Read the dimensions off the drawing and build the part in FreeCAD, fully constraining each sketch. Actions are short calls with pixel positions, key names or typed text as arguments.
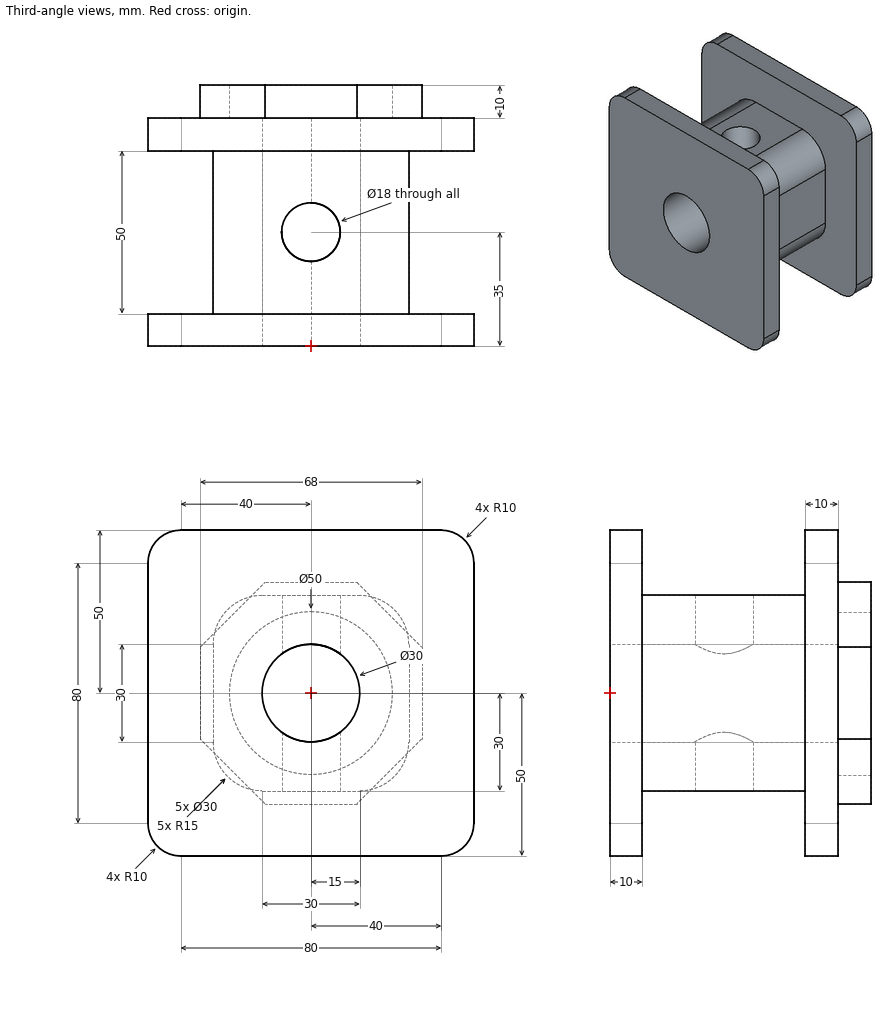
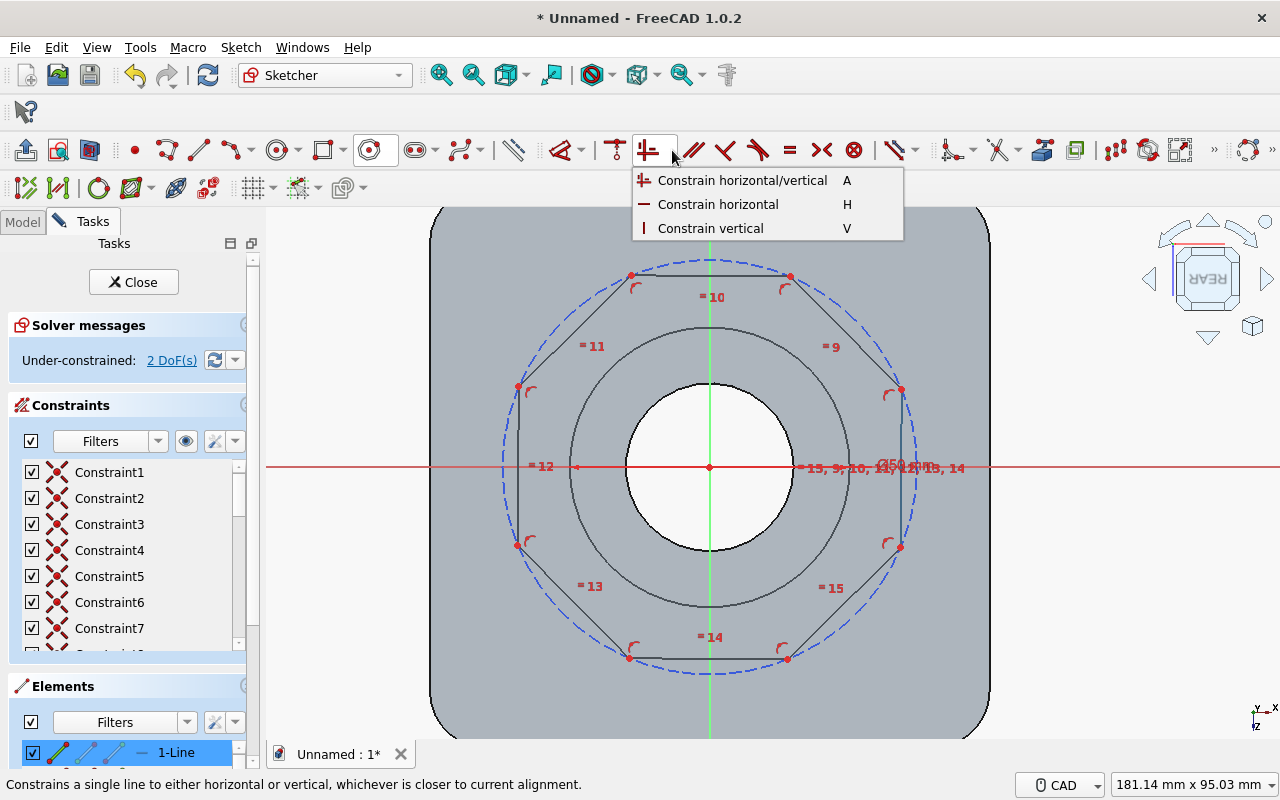
click(768, 228)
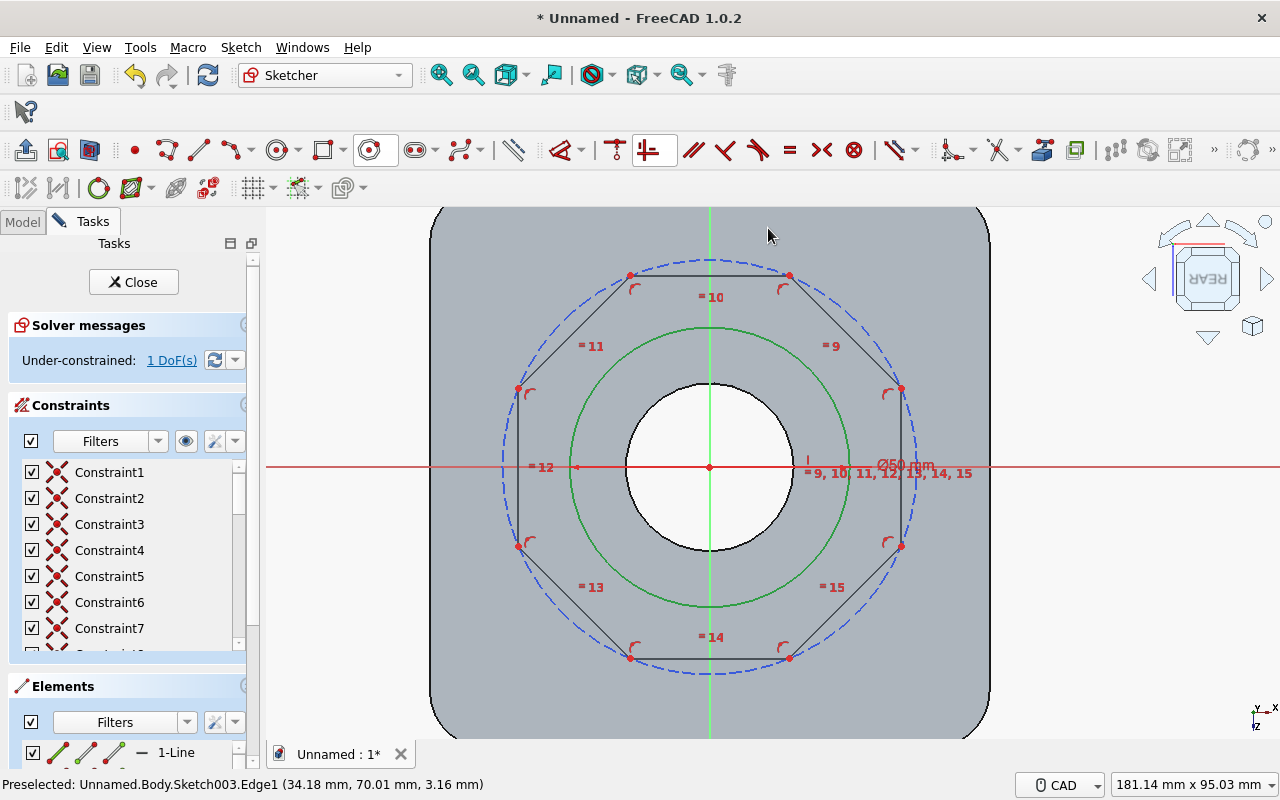
click(560, 150)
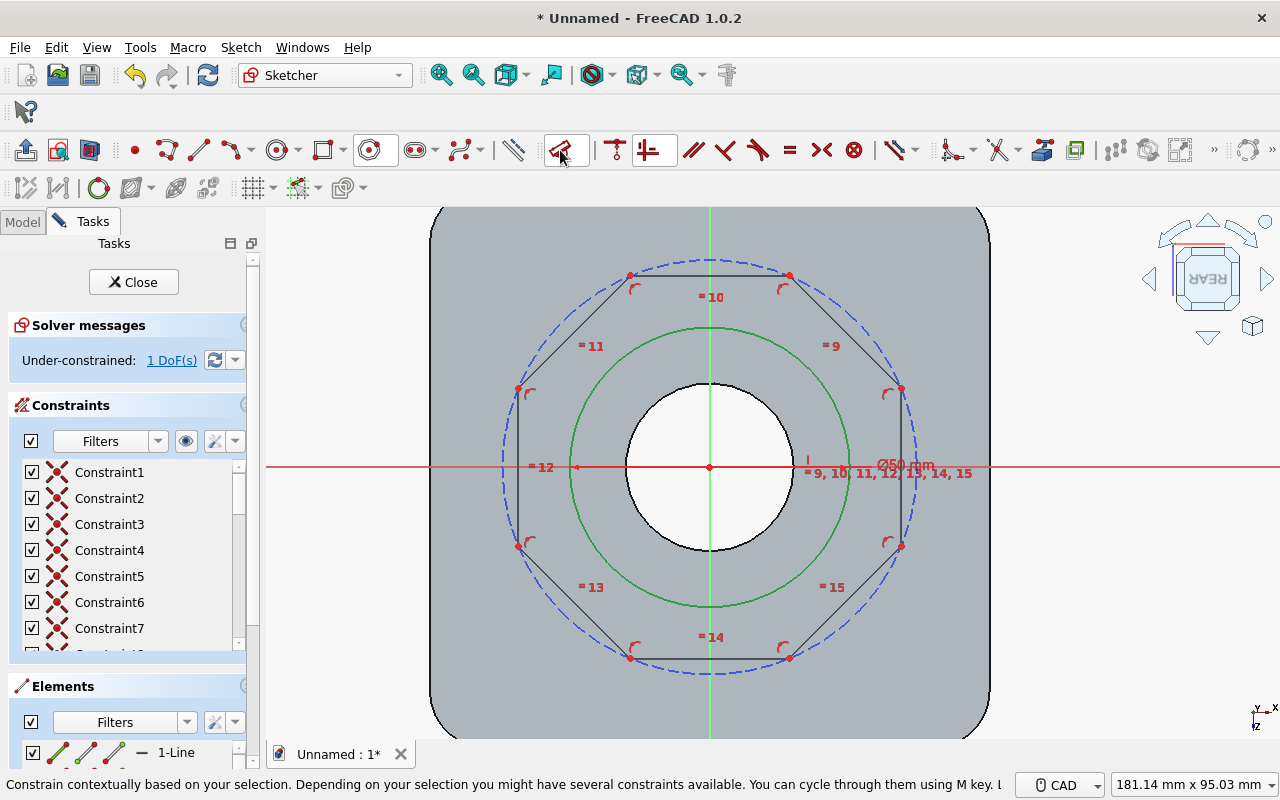
click(518, 388)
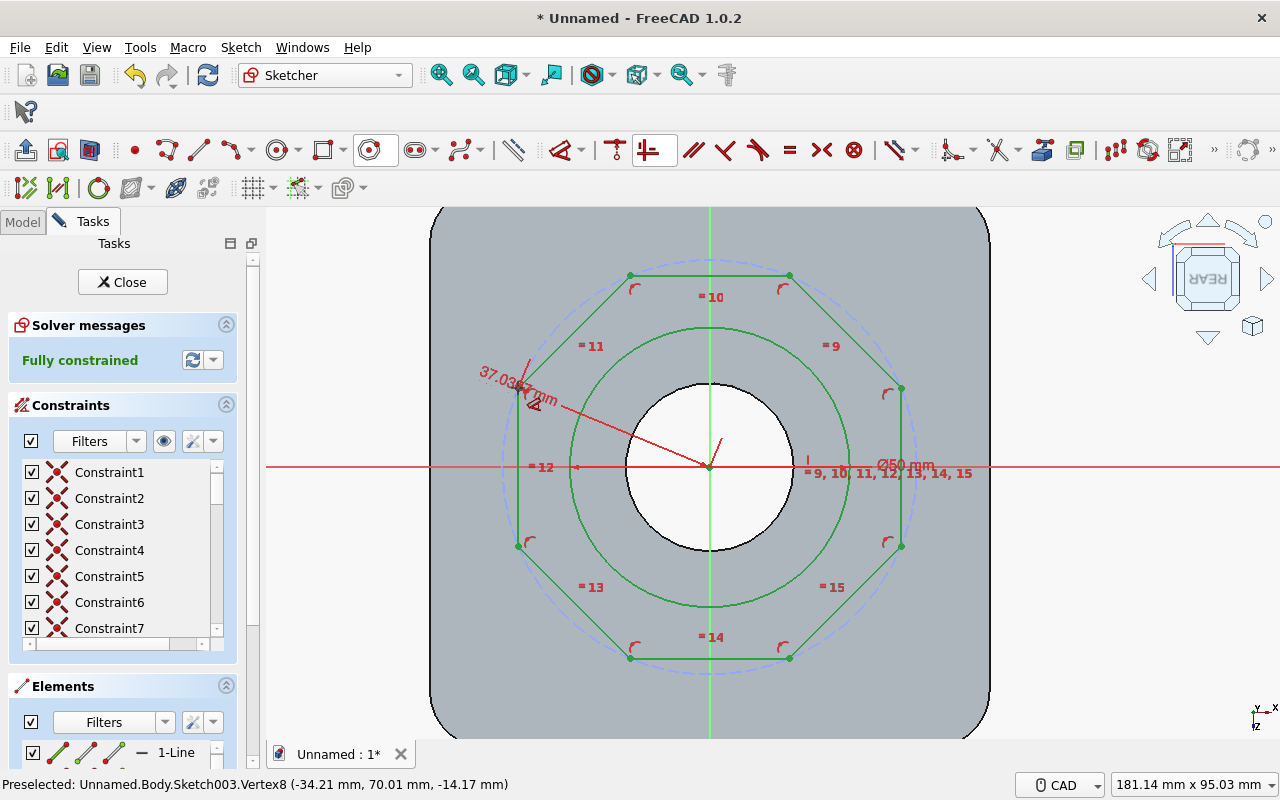
click(901, 547)
click(576, 581)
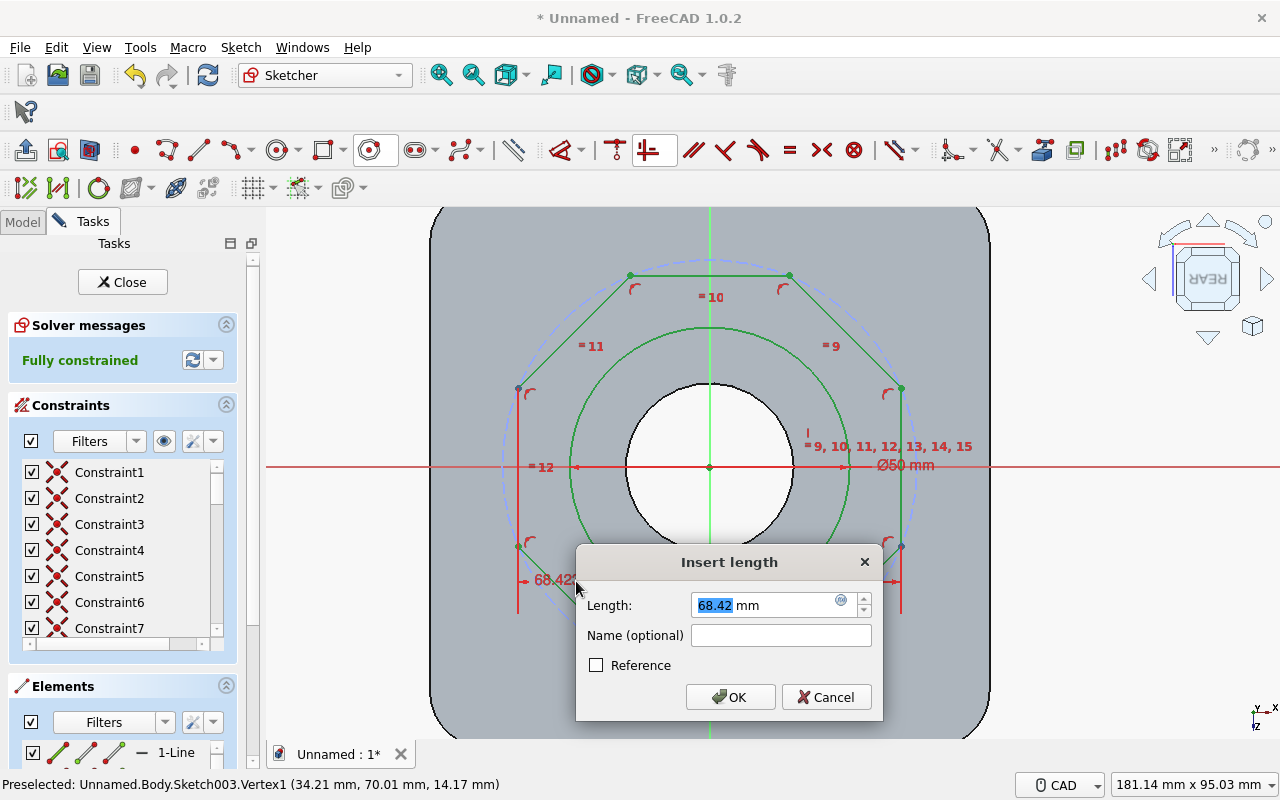
text(68)
key(Return)
key(Escape)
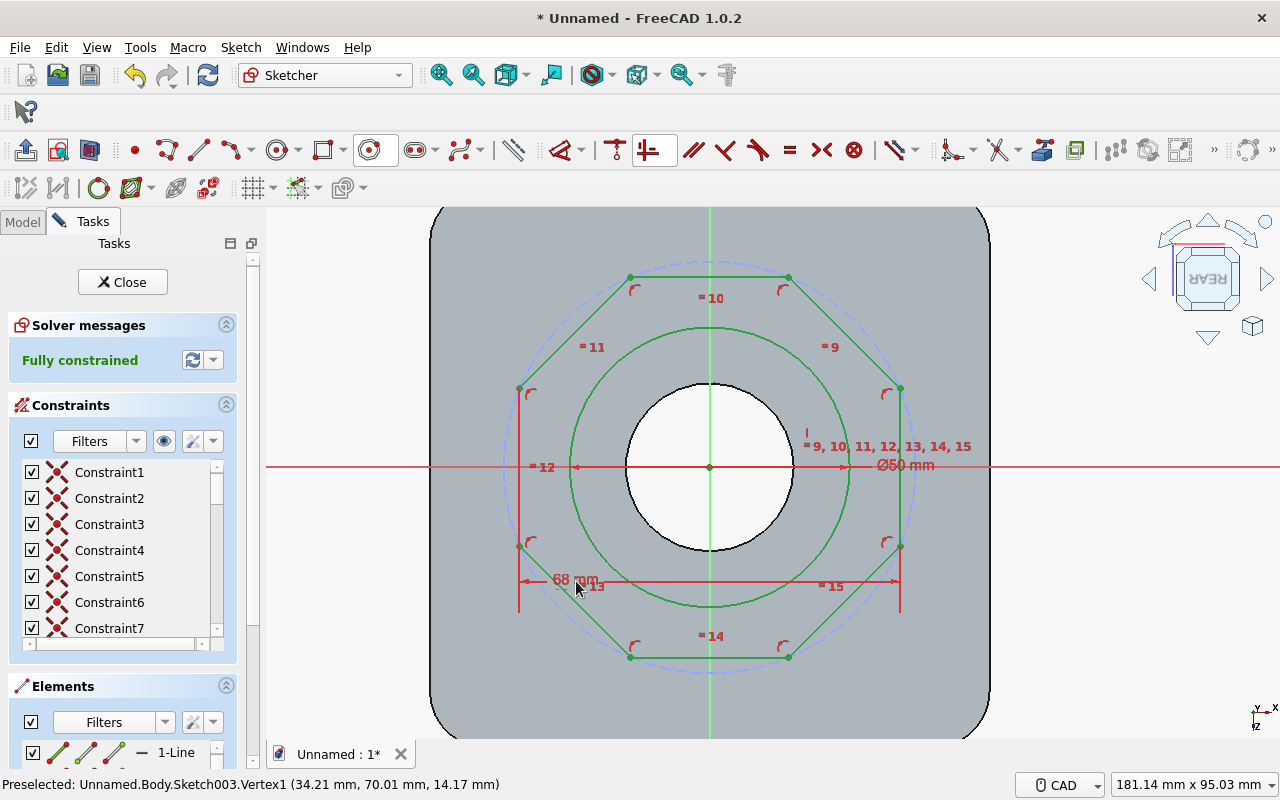
click(123, 282)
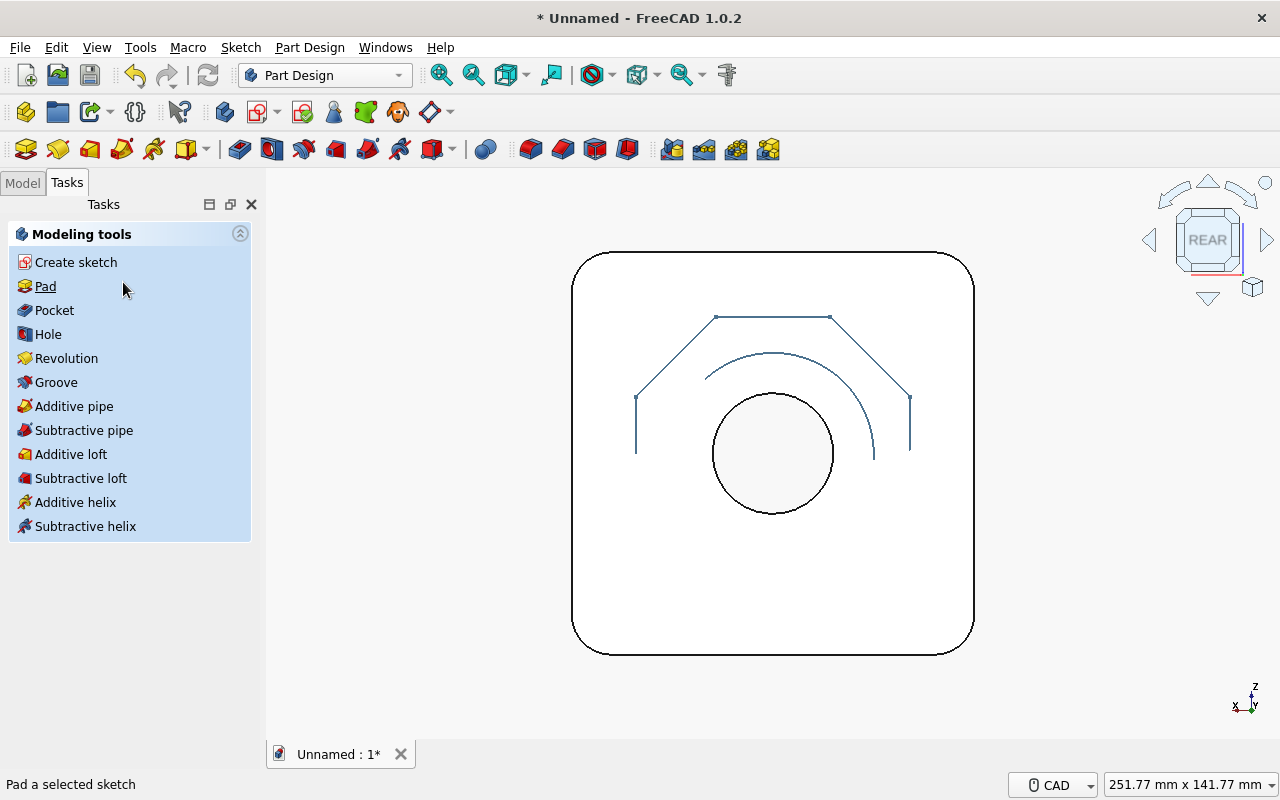
click(26, 150)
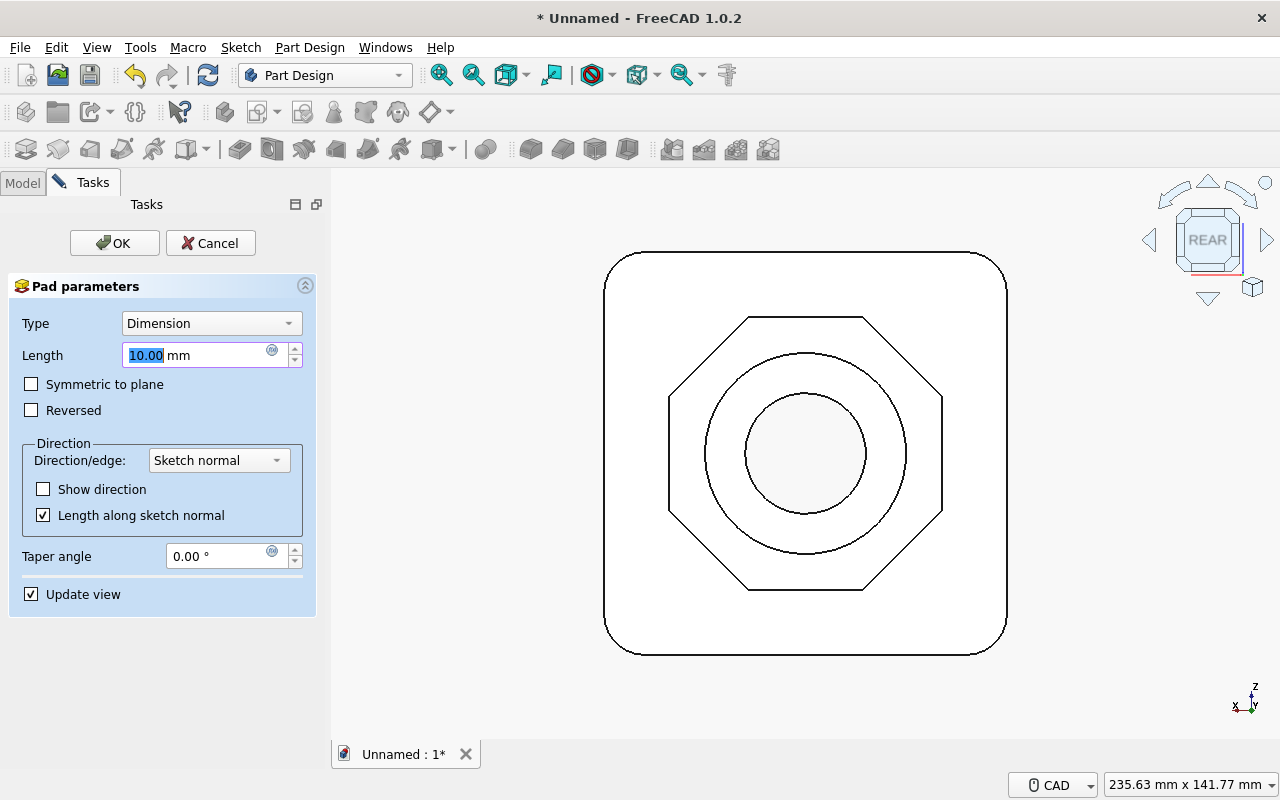
text(10)
key(Tab)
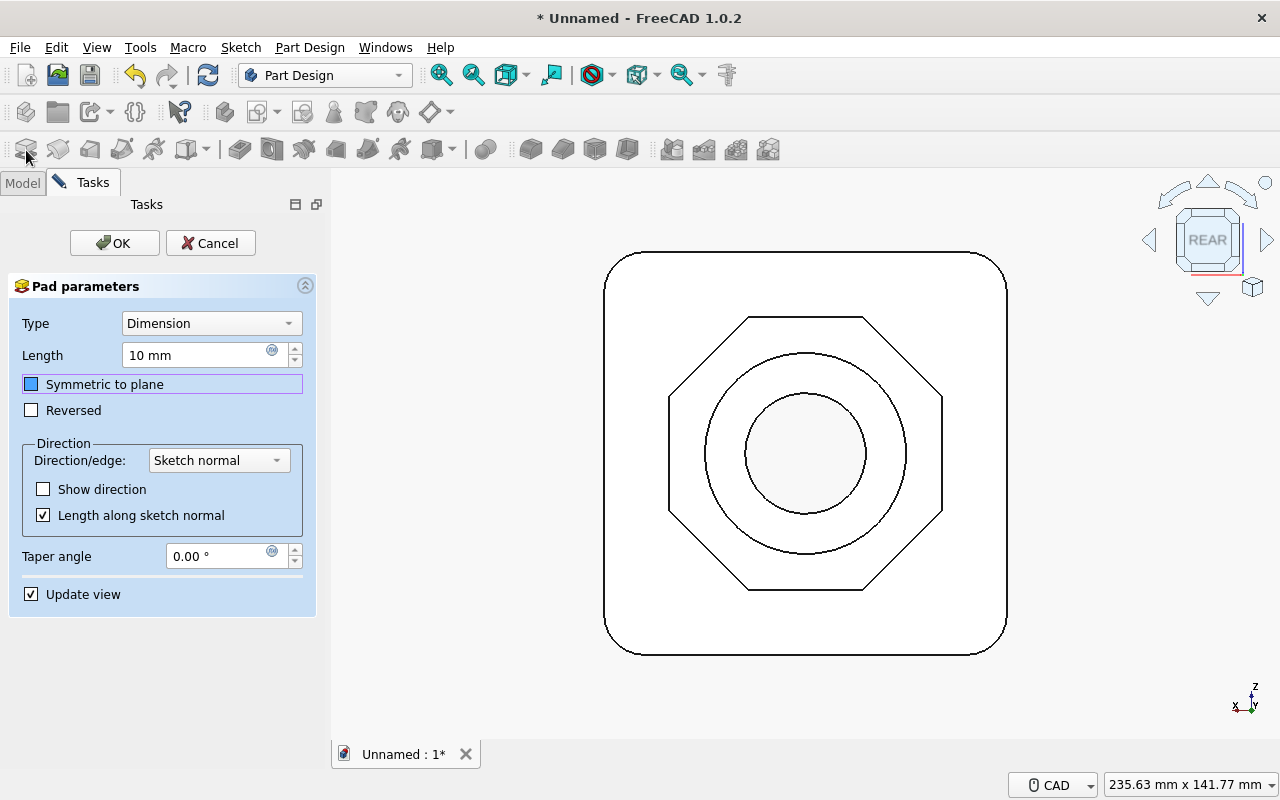
click(115, 243)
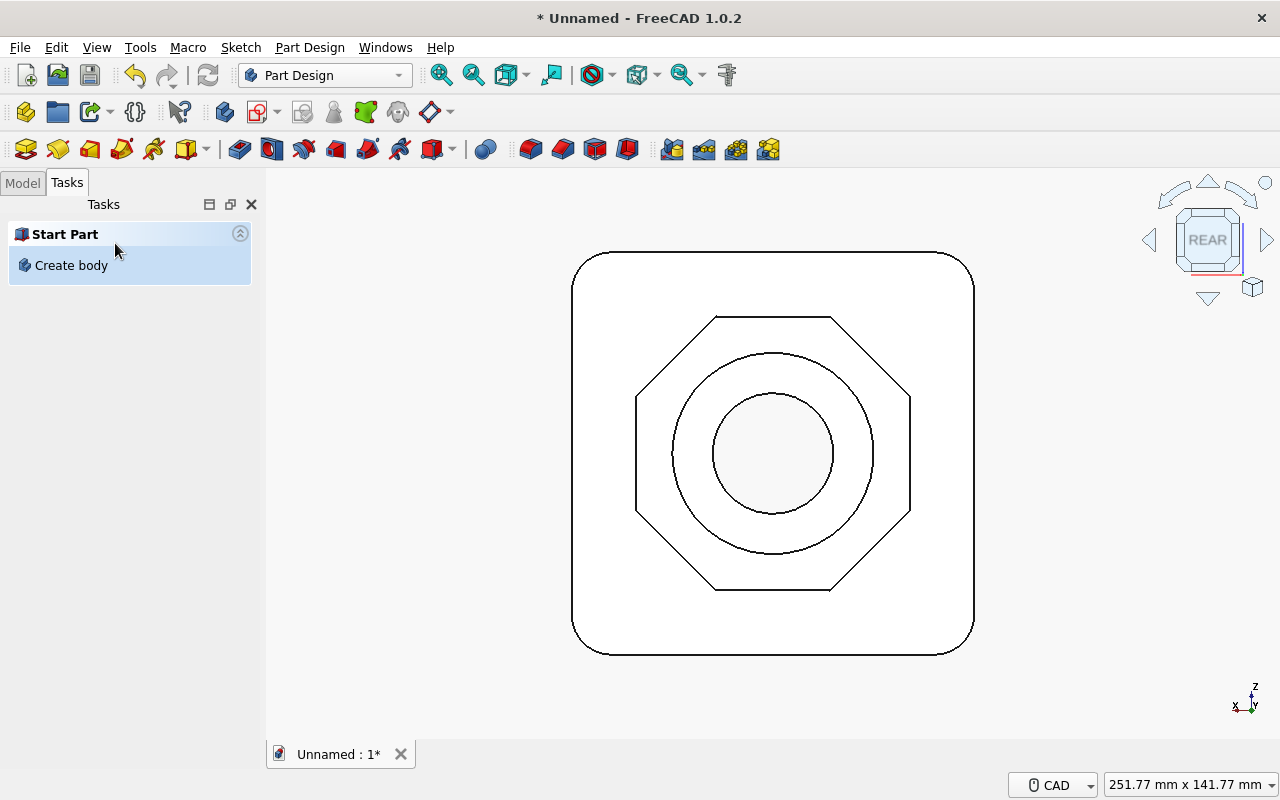
key(0)